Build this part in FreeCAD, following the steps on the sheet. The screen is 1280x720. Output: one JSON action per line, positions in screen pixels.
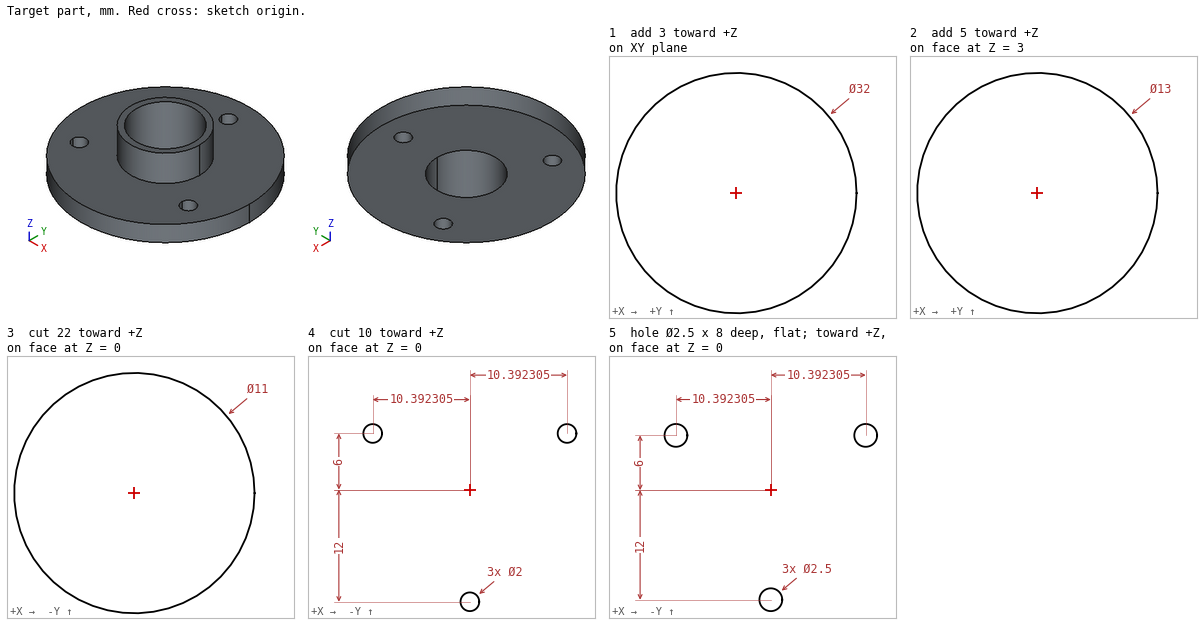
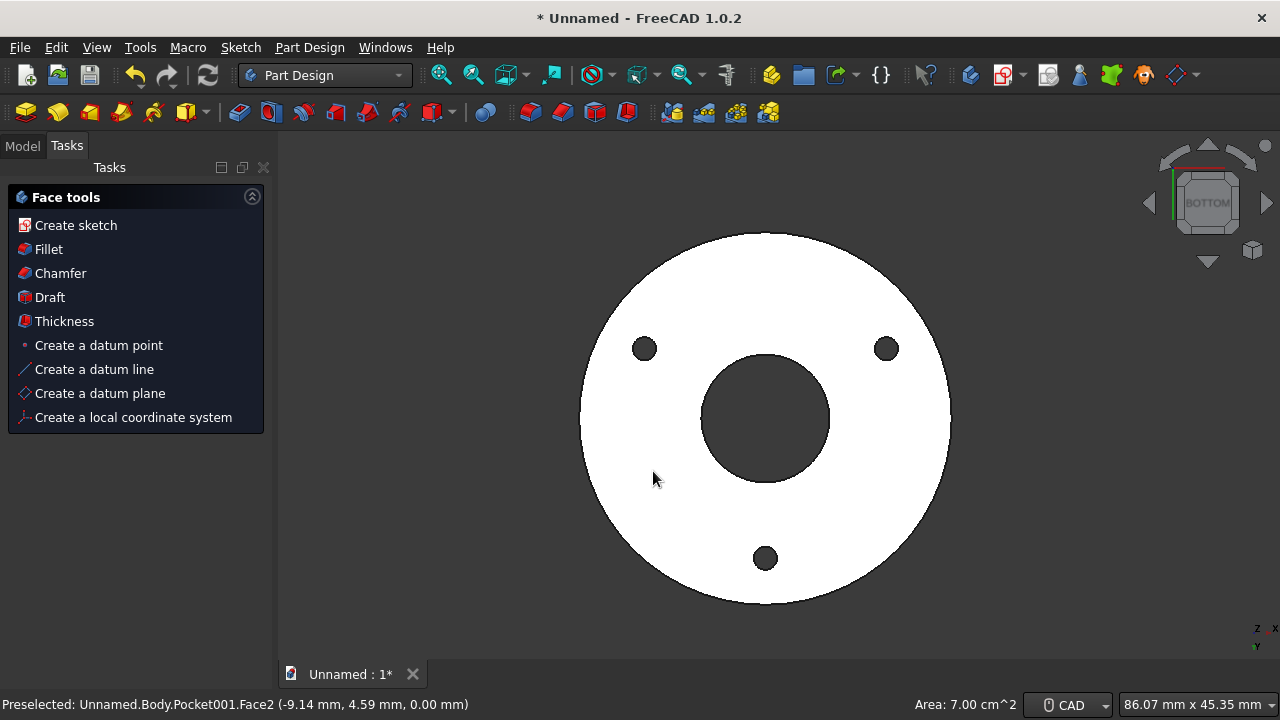
{"action": "left_click", "coordinate": [1004, 76]}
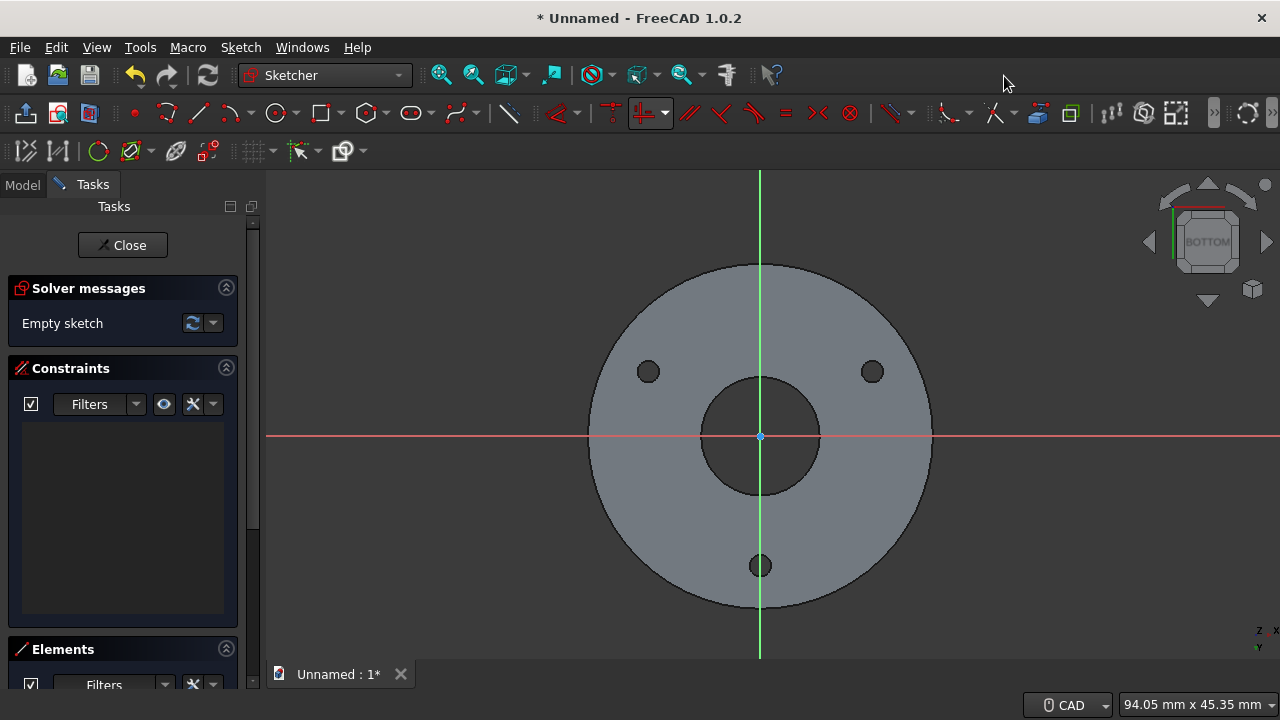
{"action": "scroll", "coordinate": [874, 579], "scroll_direction": "up", "scroll_amount": 2}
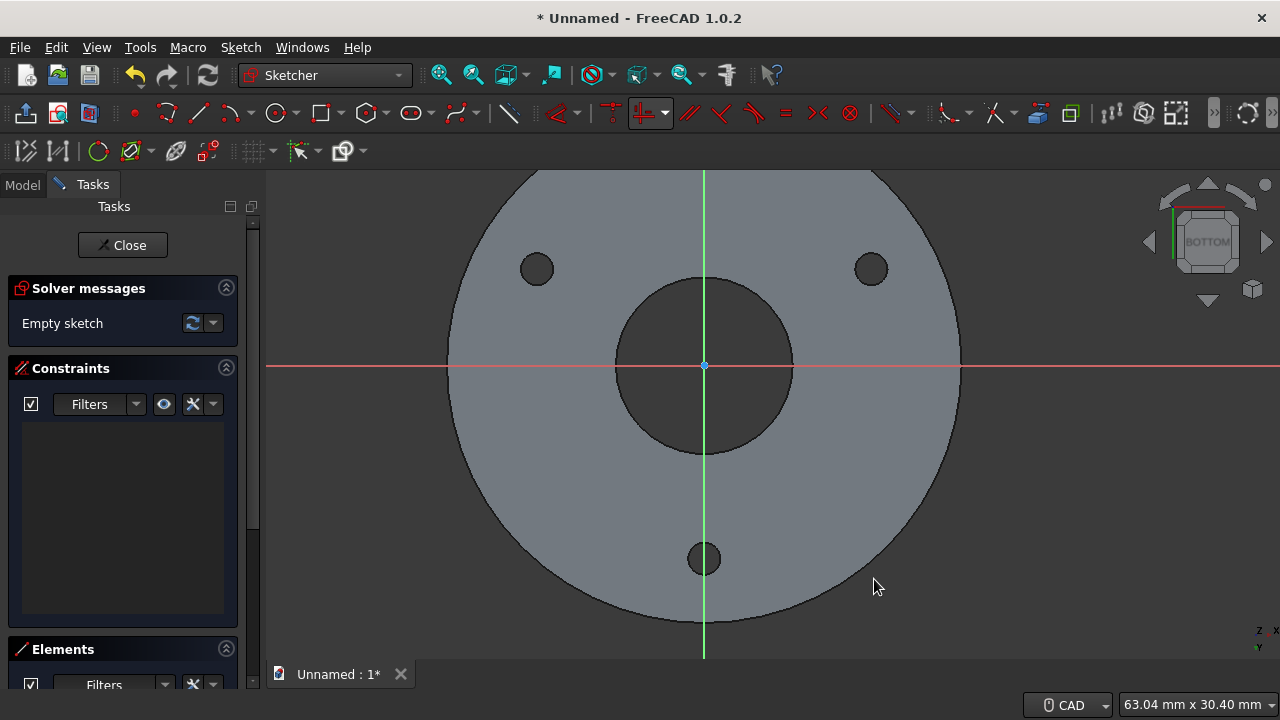
{"action": "left_click", "coordinate": [276, 114]}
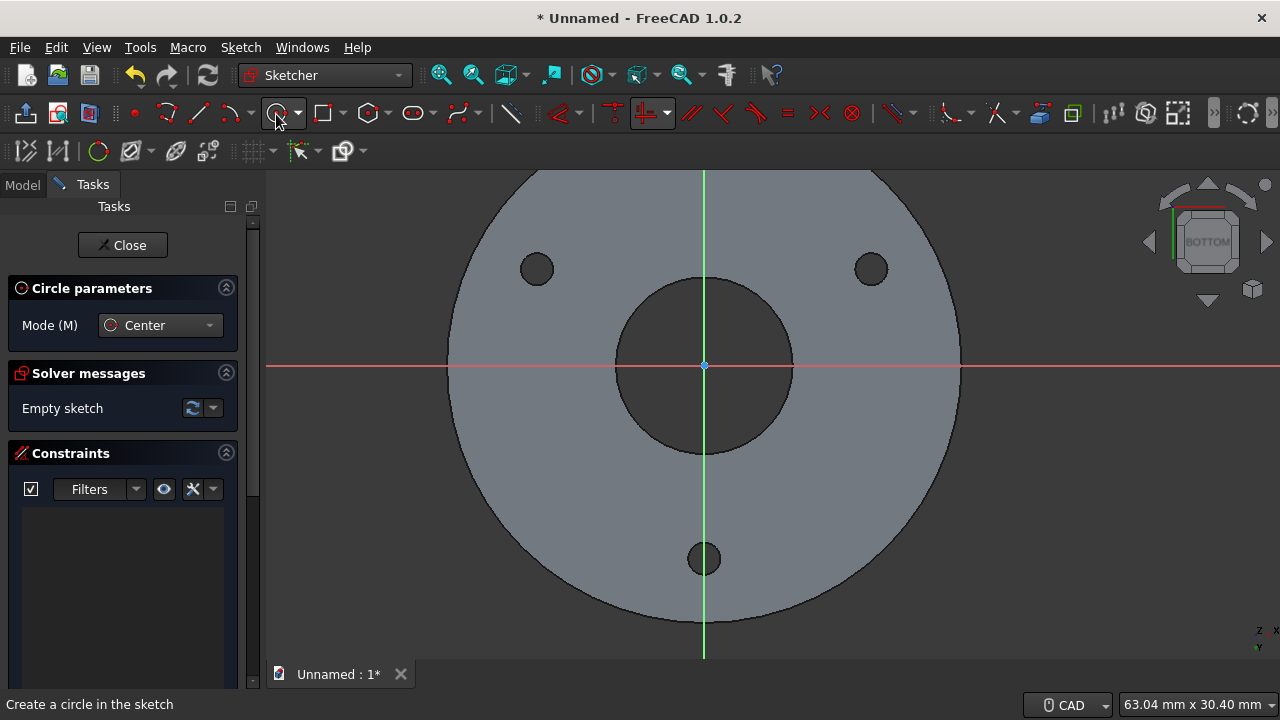
{"action": "left_click", "coordinate": [704, 559]}
{"action": "mouse_move", "coordinate": [718, 545]}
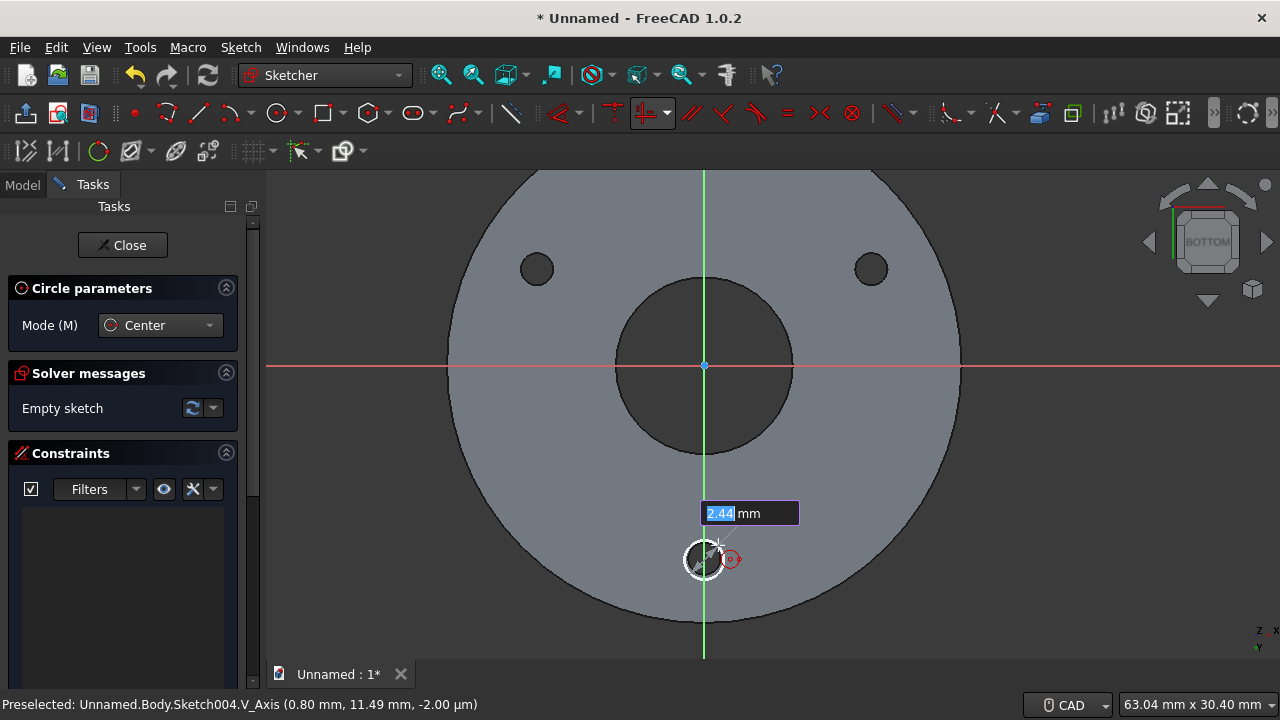
{"action": "type", "text": "2.5"}
{"action": "key", "text": "Return"}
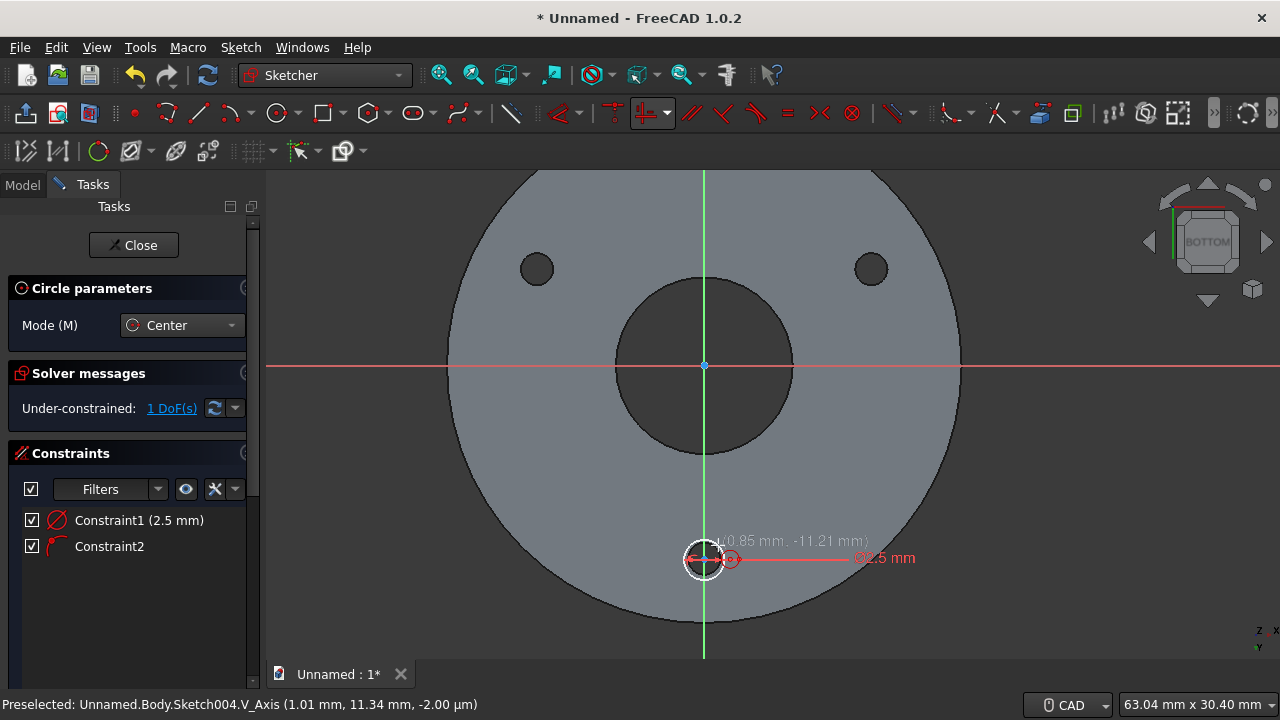
{"action": "left_click", "coordinate": [537, 269]}
{"action": "mouse_move", "coordinate": [551, 255]}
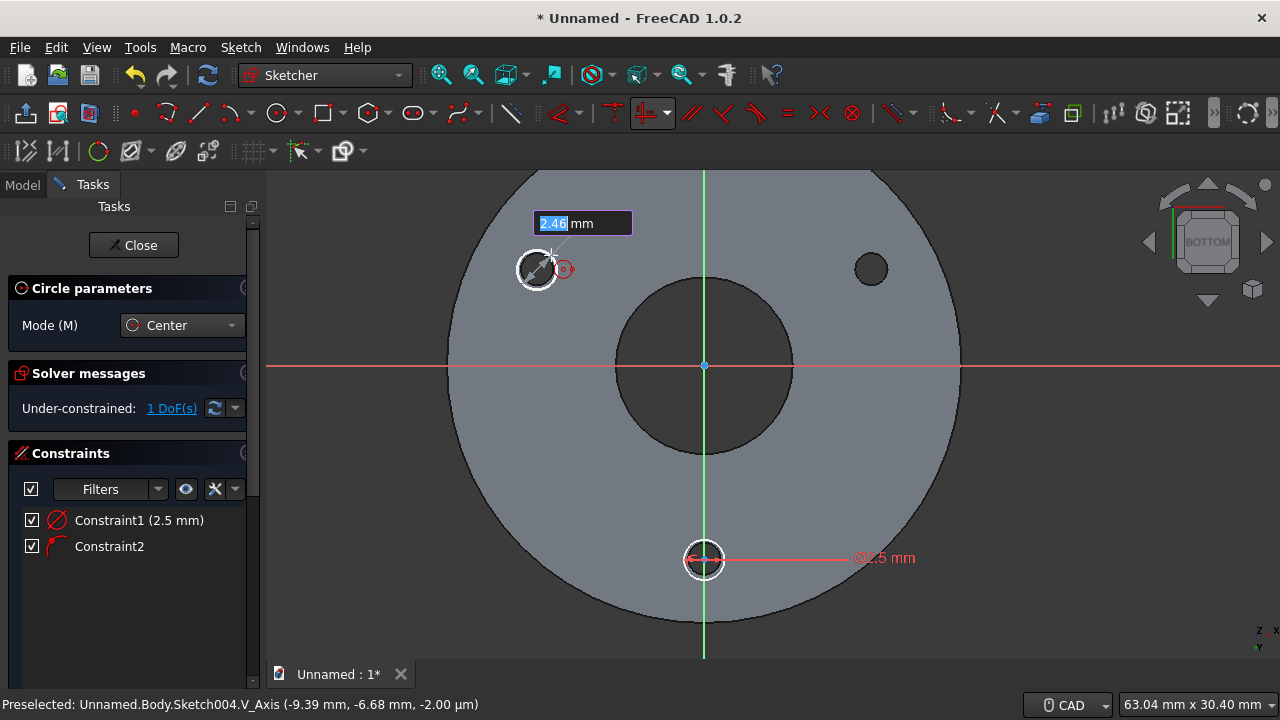
{"action": "type", "text": "2.5"}
{"action": "key", "text": "Return"}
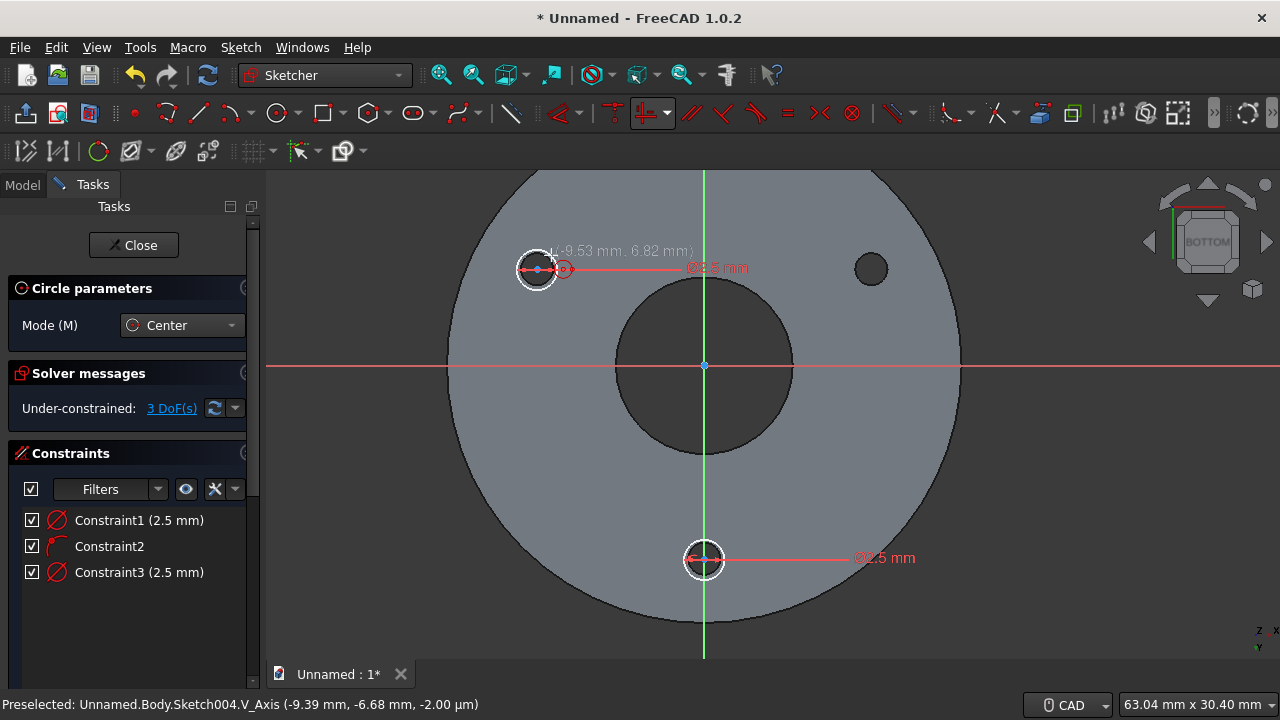
{"action": "left_click", "coordinate": [871, 269]}
{"action": "mouse_move", "coordinate": [886, 255]}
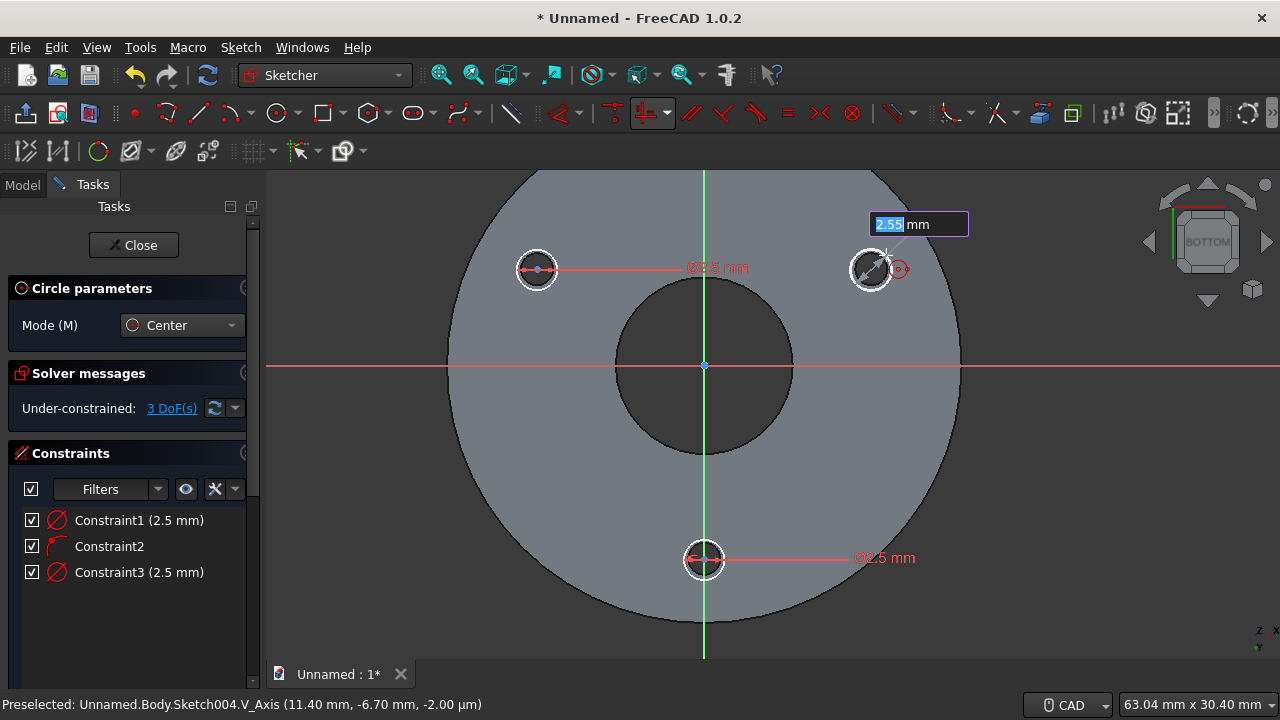
{"action": "type", "text": "2.5"}
{"action": "key", "text": "Return"}
{"action": "key", "text": "Escape"}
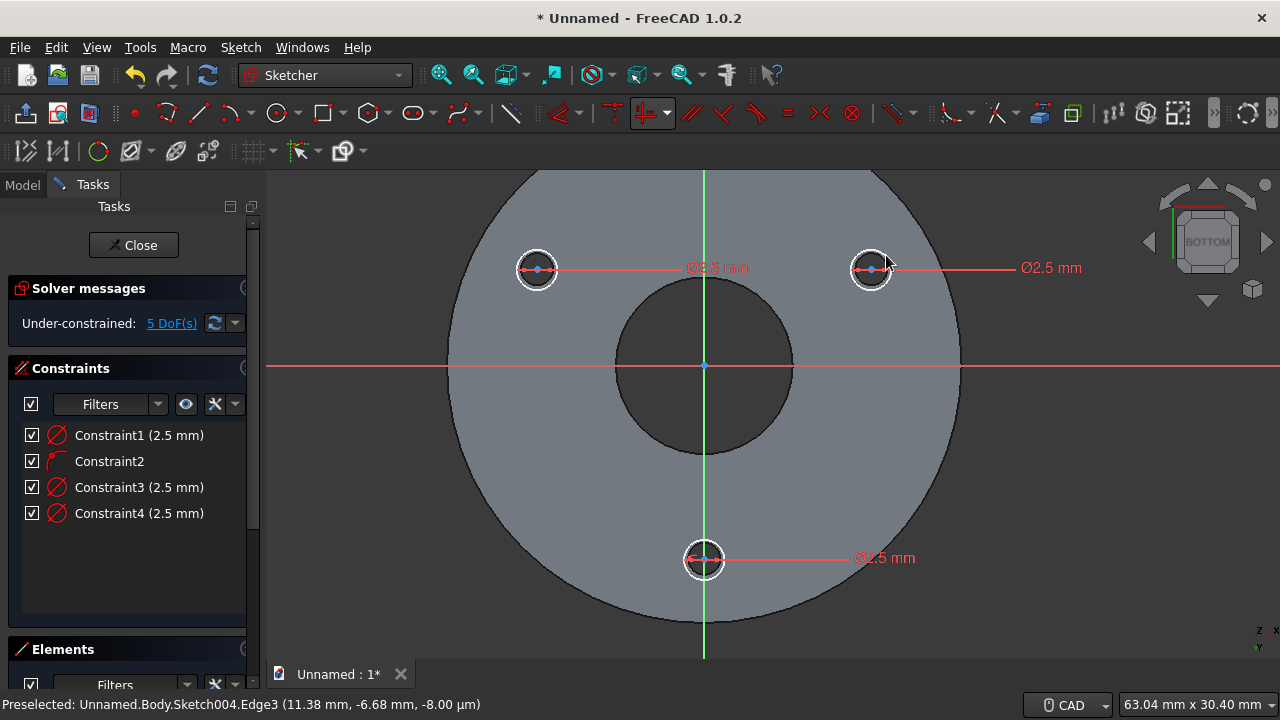
{"action": "left_click", "coordinate": [537, 270]}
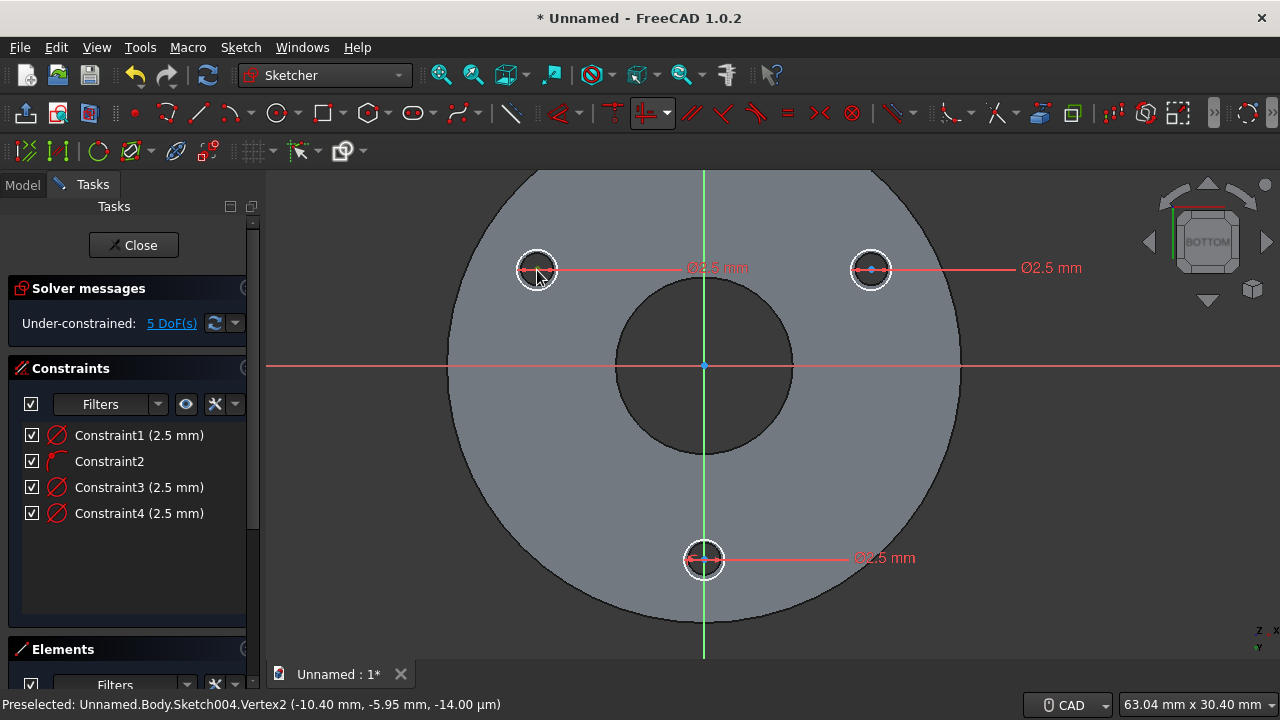
{"action": "left_click", "coordinate": [871, 270]}